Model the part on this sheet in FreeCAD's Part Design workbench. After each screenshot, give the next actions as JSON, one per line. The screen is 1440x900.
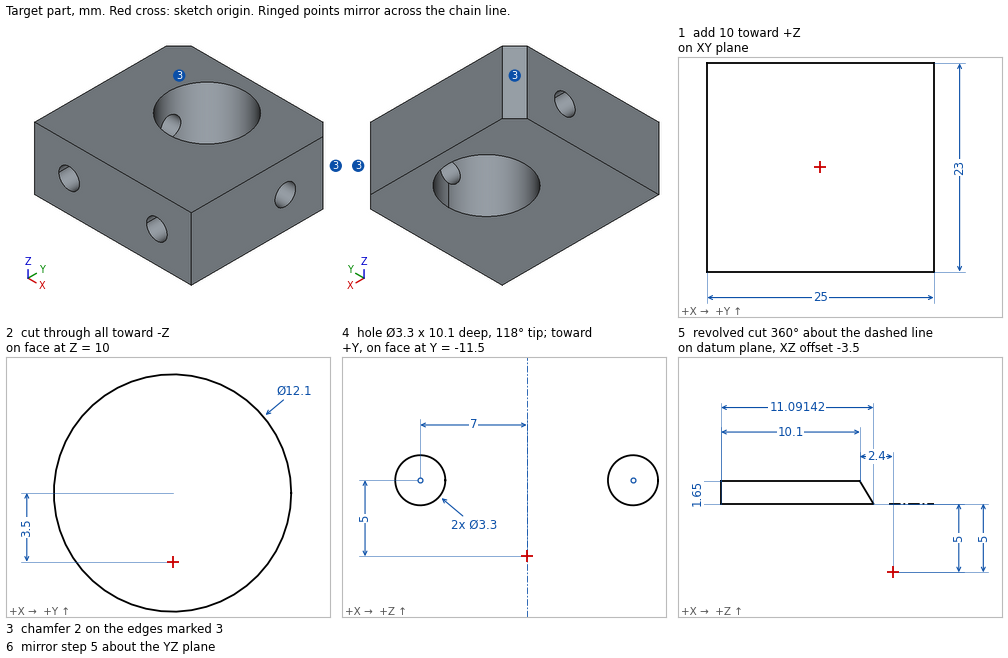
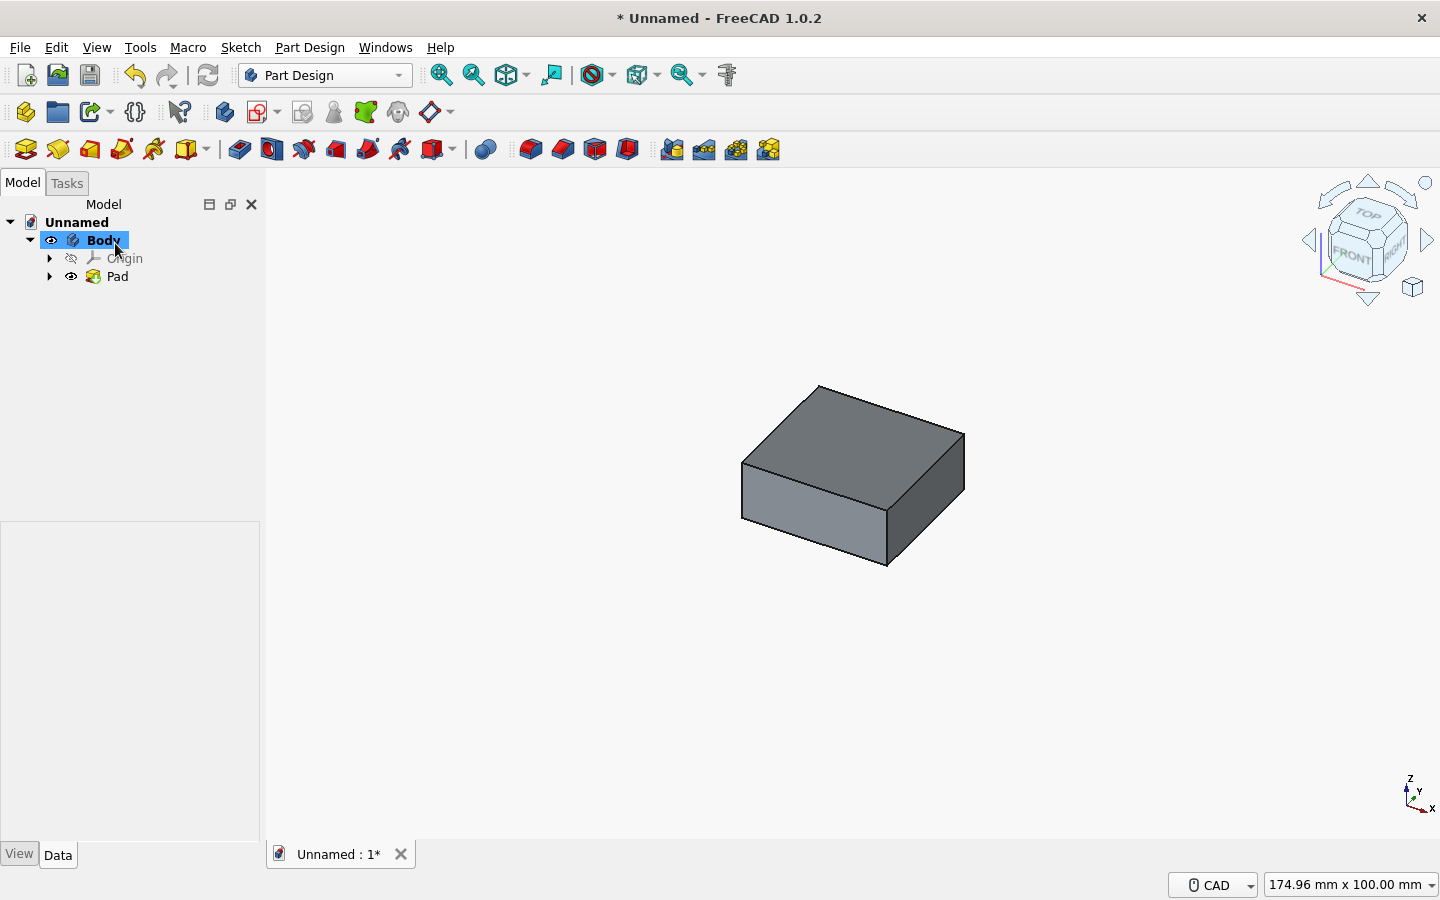
{"action": "left_click", "coordinate": [442, 76]}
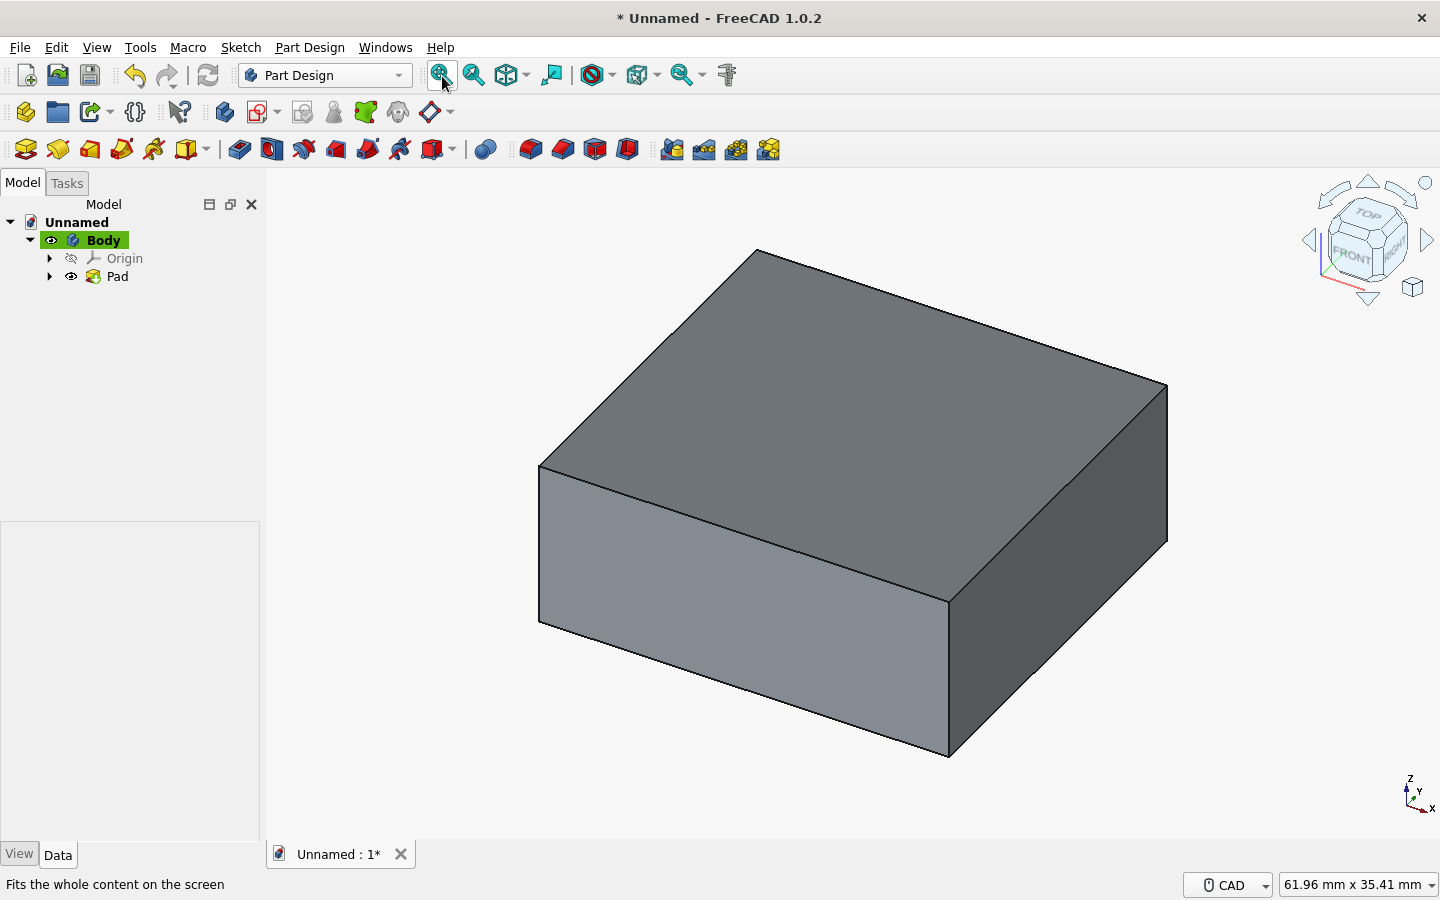
{"action": "left_click", "coordinate": [853, 425]}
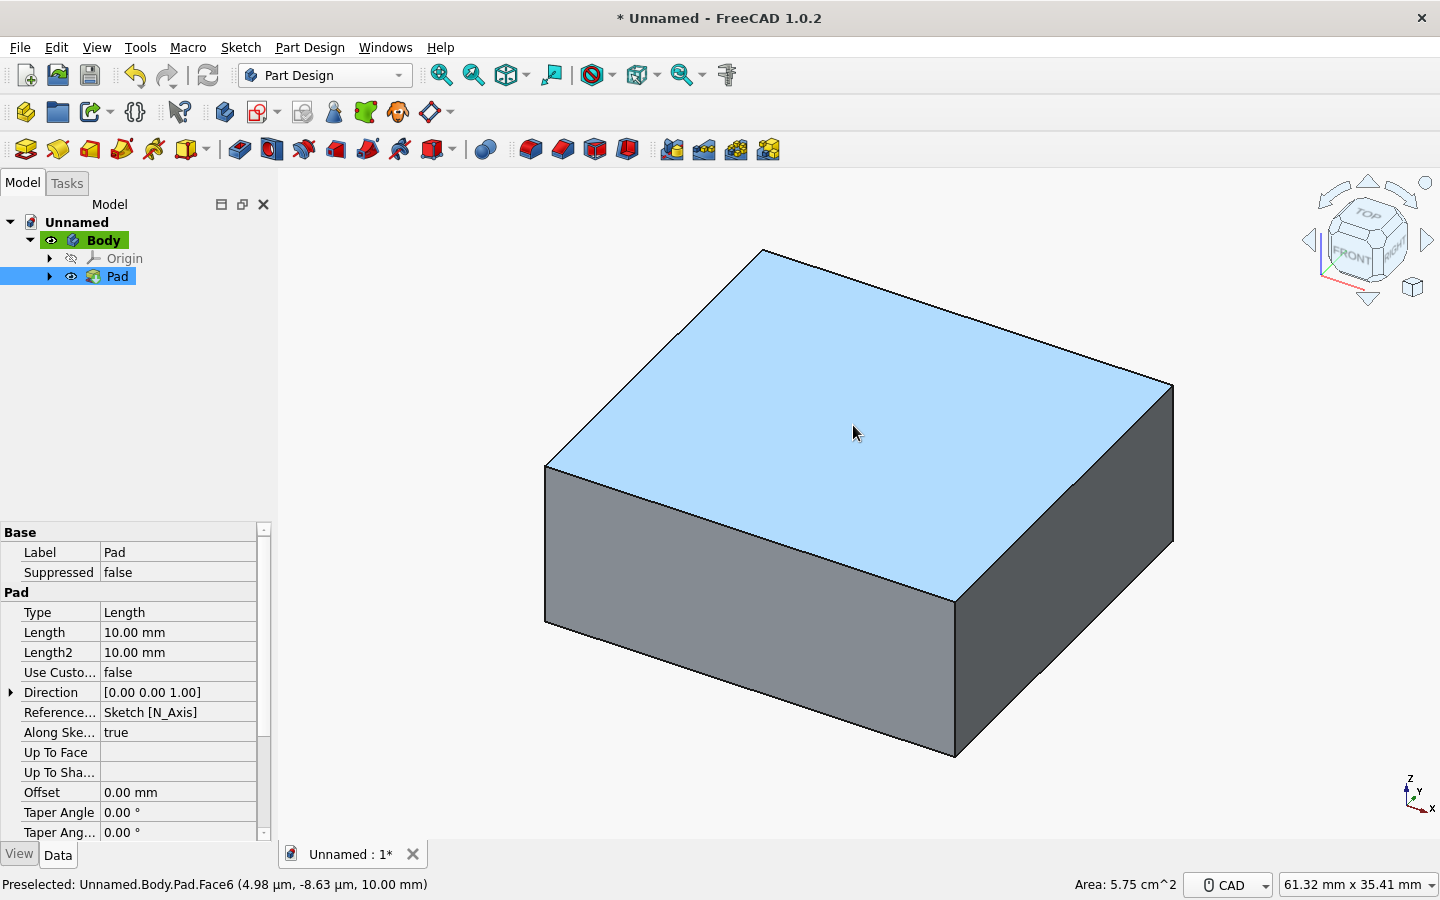
{"action": "left_click", "coordinate": [258, 112]}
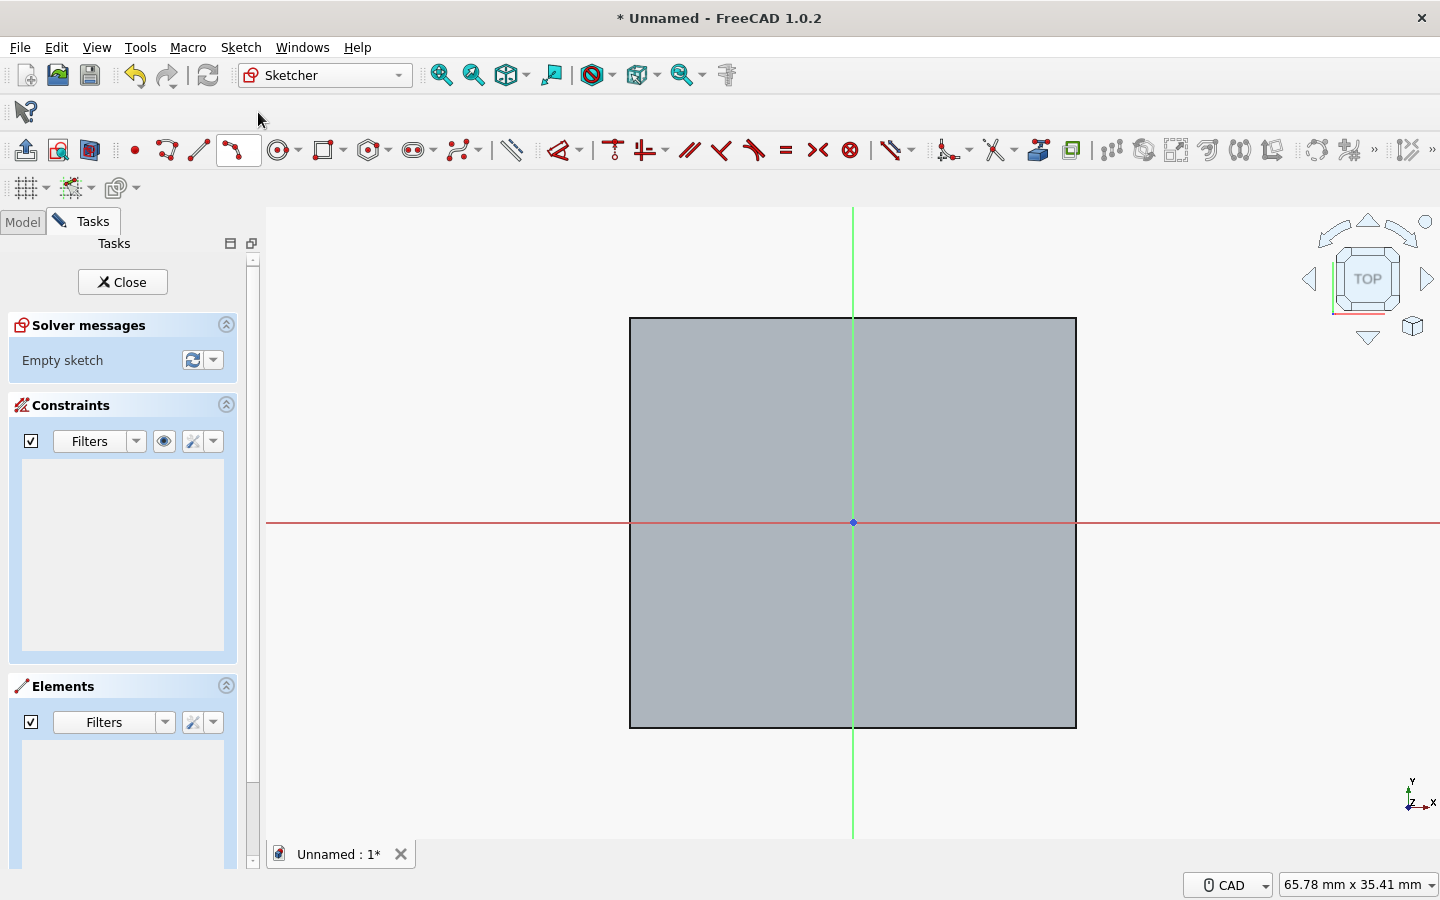
{"action": "scroll", "coordinate": [936, 385], "scroll_direction": "up", "scroll_amount": 3}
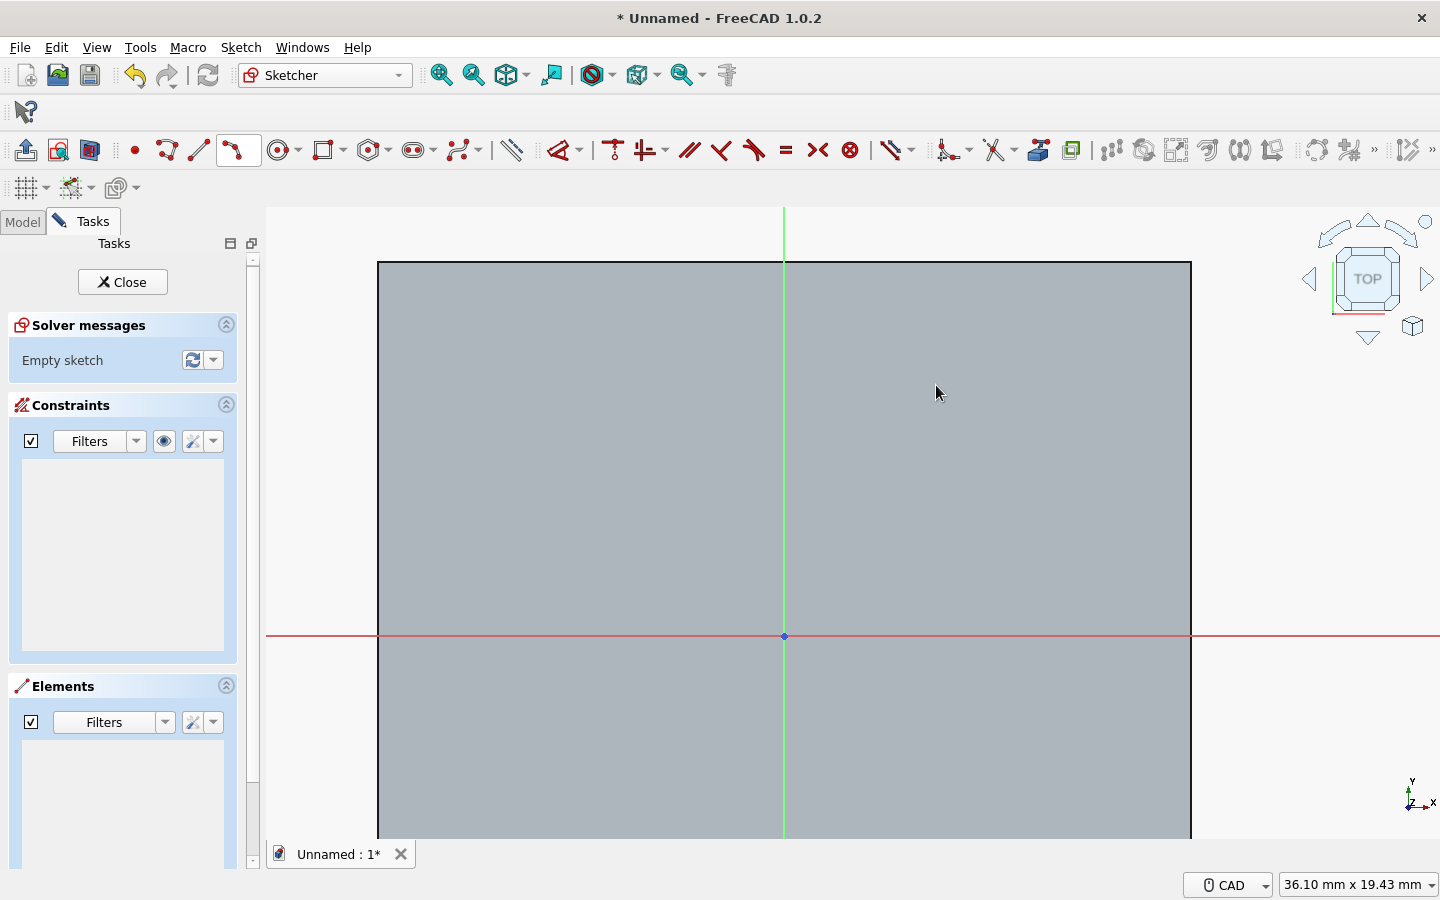
{"action": "left_click", "coordinate": [278, 150]}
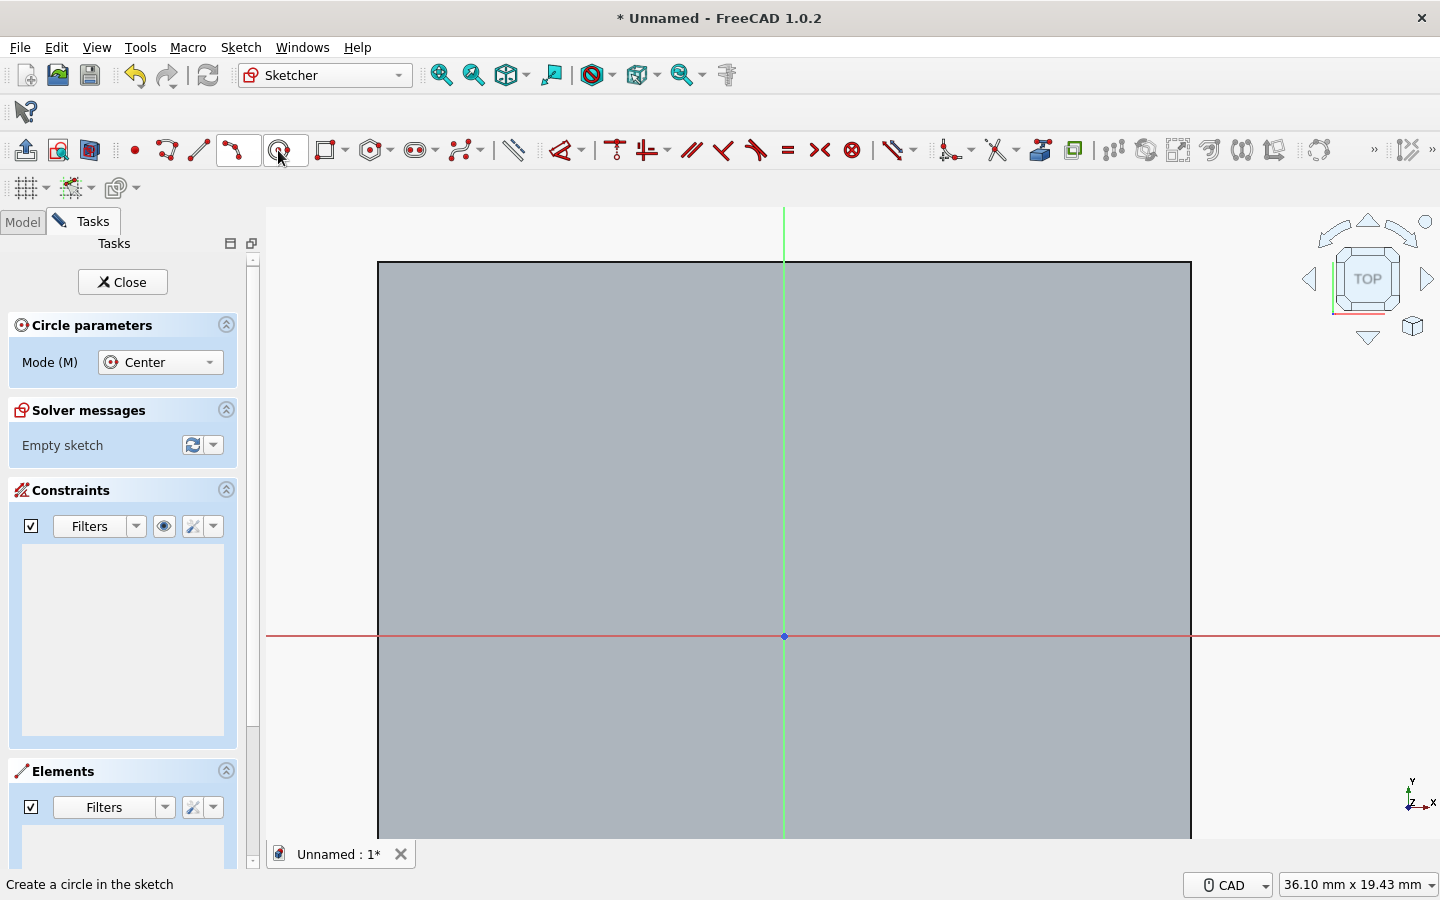
{"action": "left_click", "coordinate": [784, 522]}
{"action": "left_click", "coordinate": [923, 383]}
{"action": "key", "text": "Escape"}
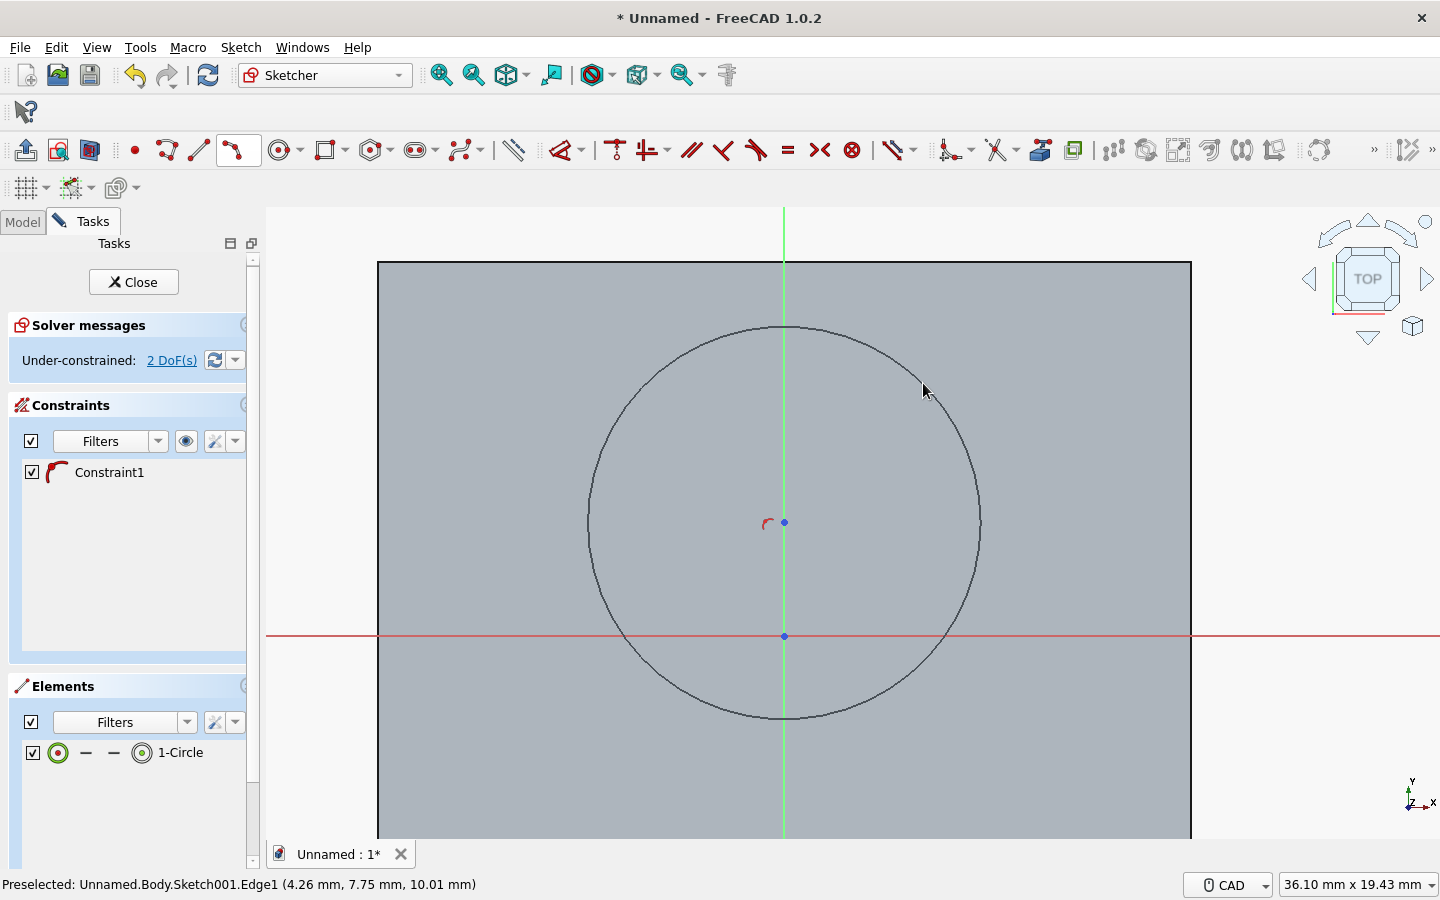
{"action": "key", "text": "d"}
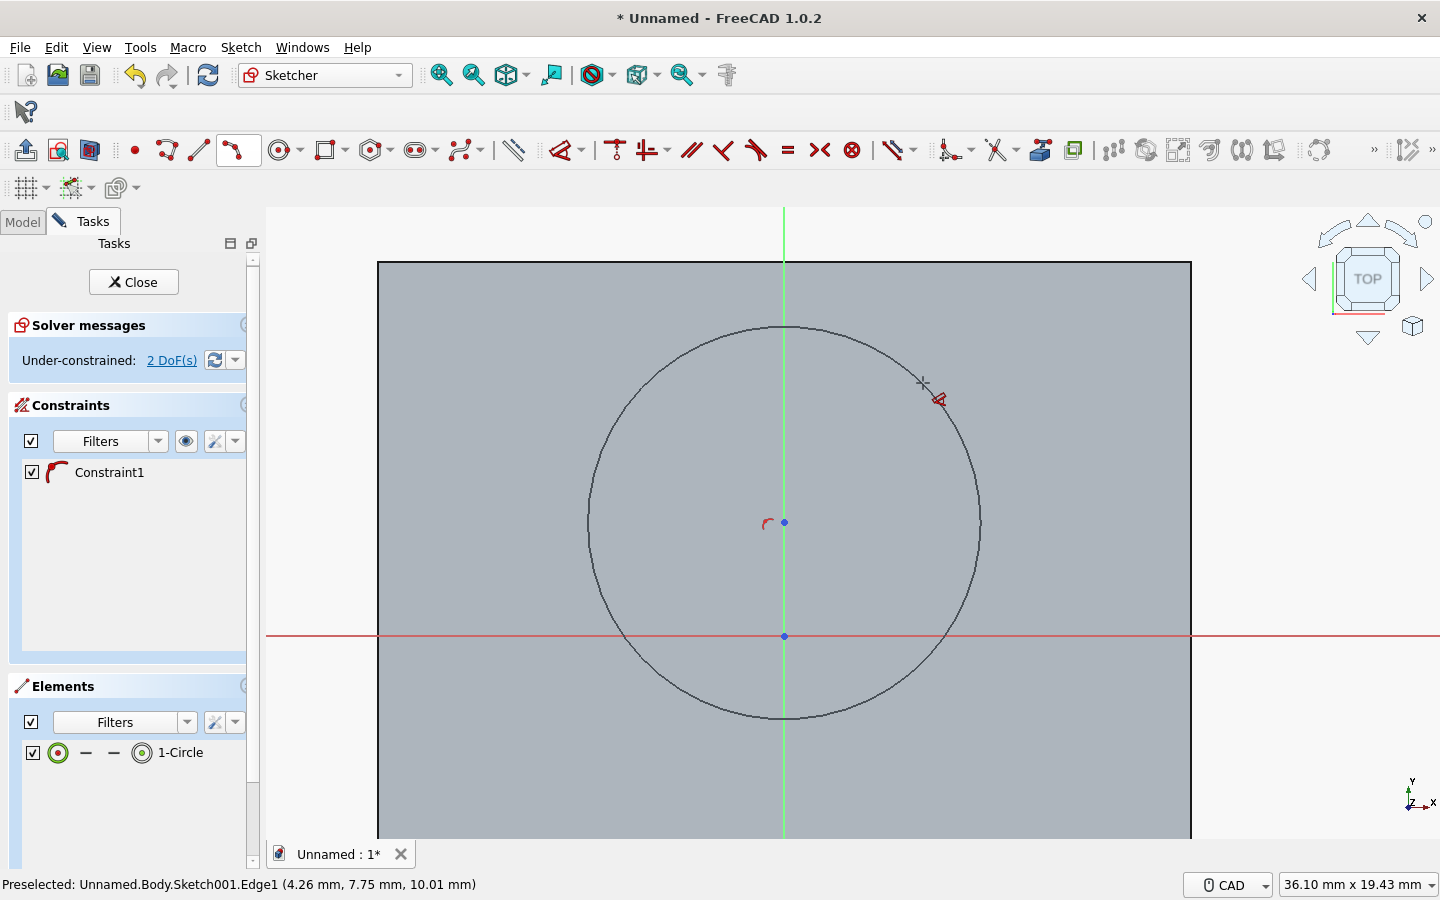
{"action": "left_click", "coordinate": [923, 384]}
{"action": "left_click", "coordinate": [946, 361]}